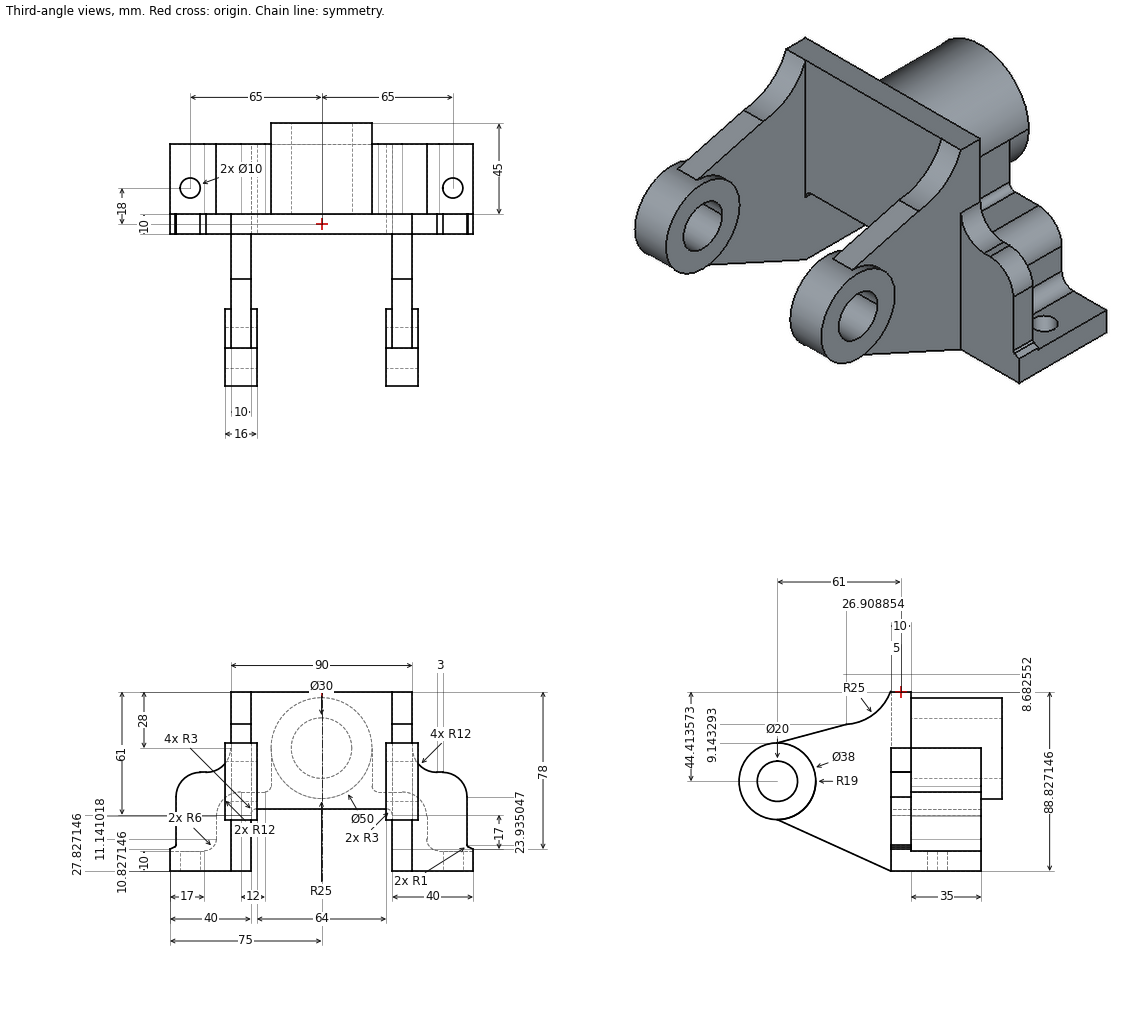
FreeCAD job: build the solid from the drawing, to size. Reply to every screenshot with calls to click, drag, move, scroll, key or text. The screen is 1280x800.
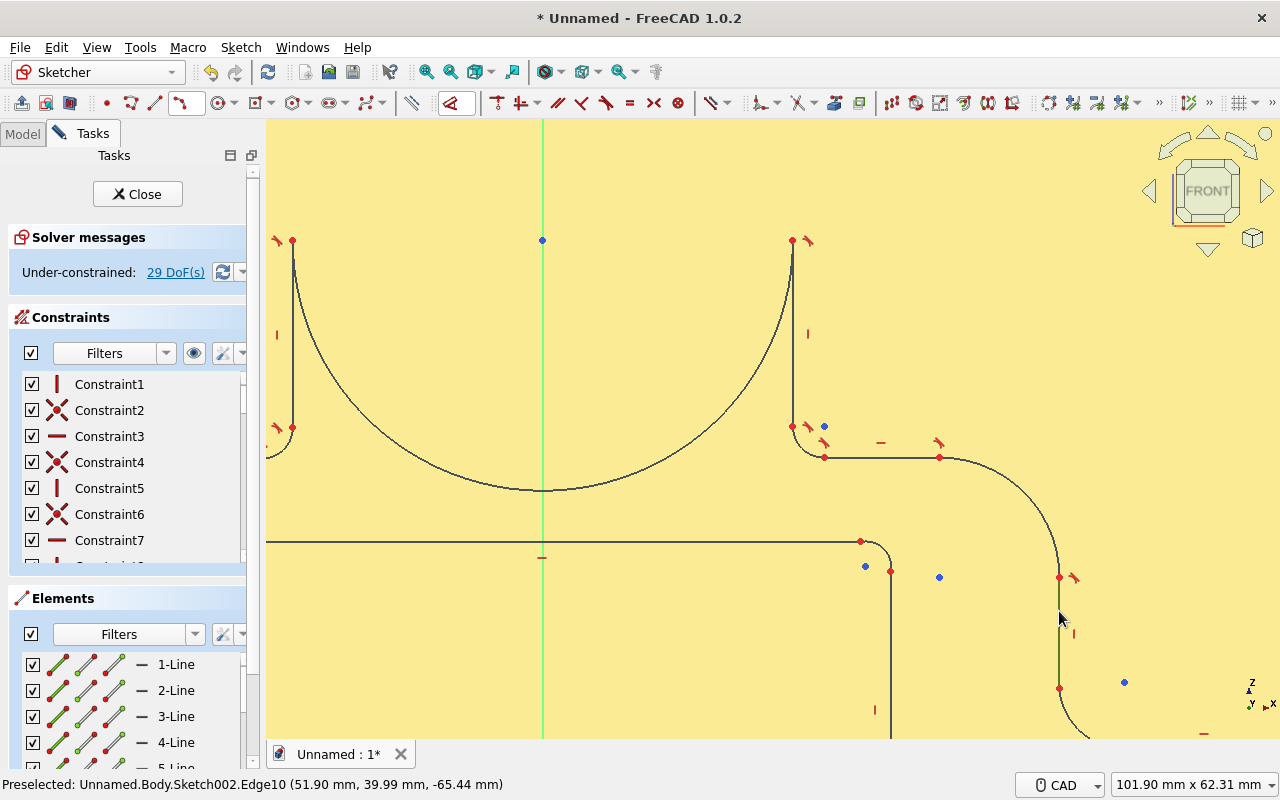
click(1063, 707)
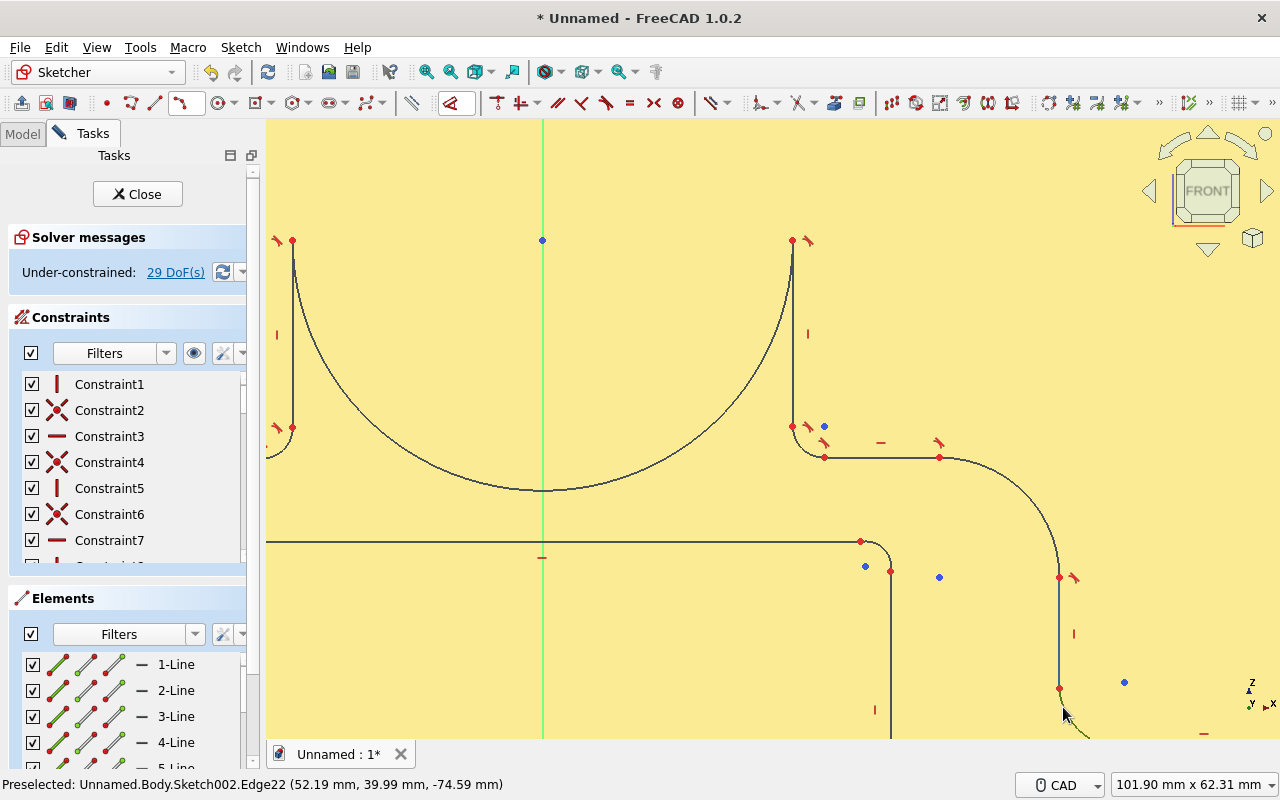
key(t)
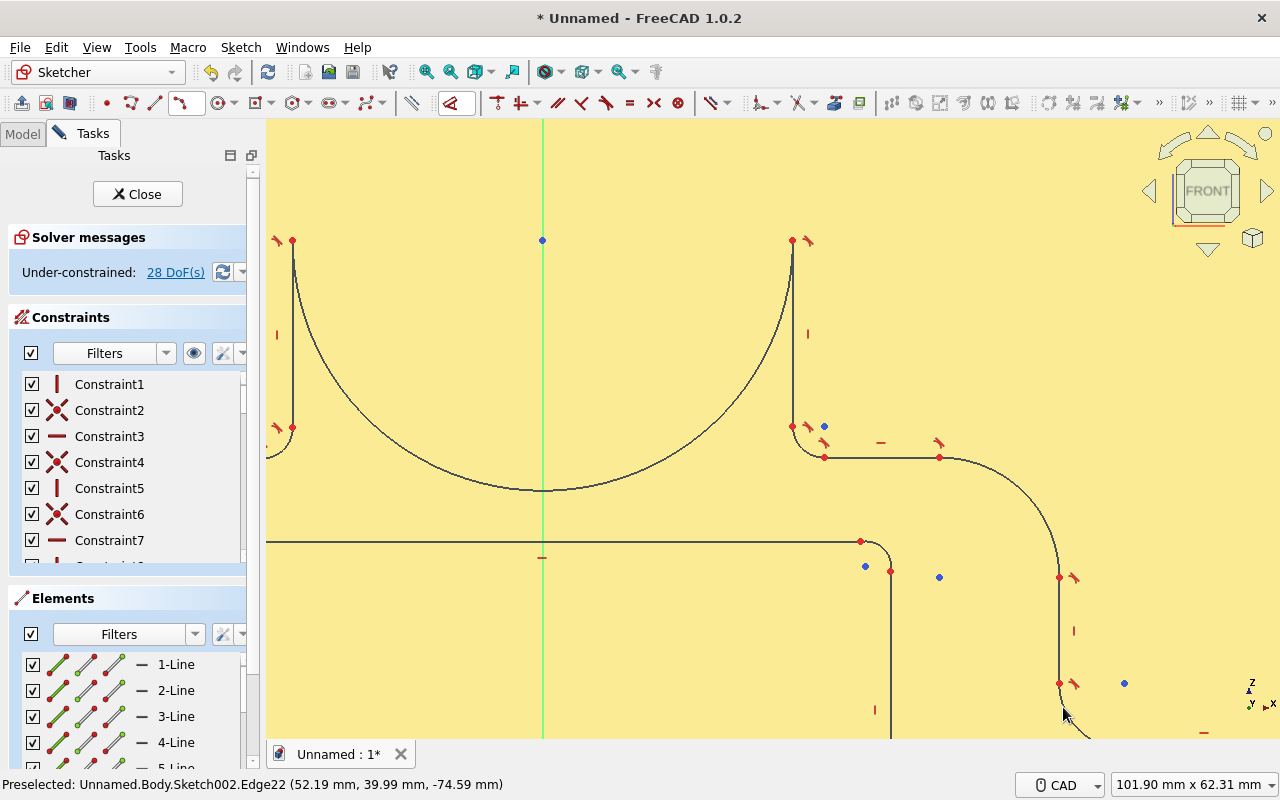
scroll(799, 444, down, 5)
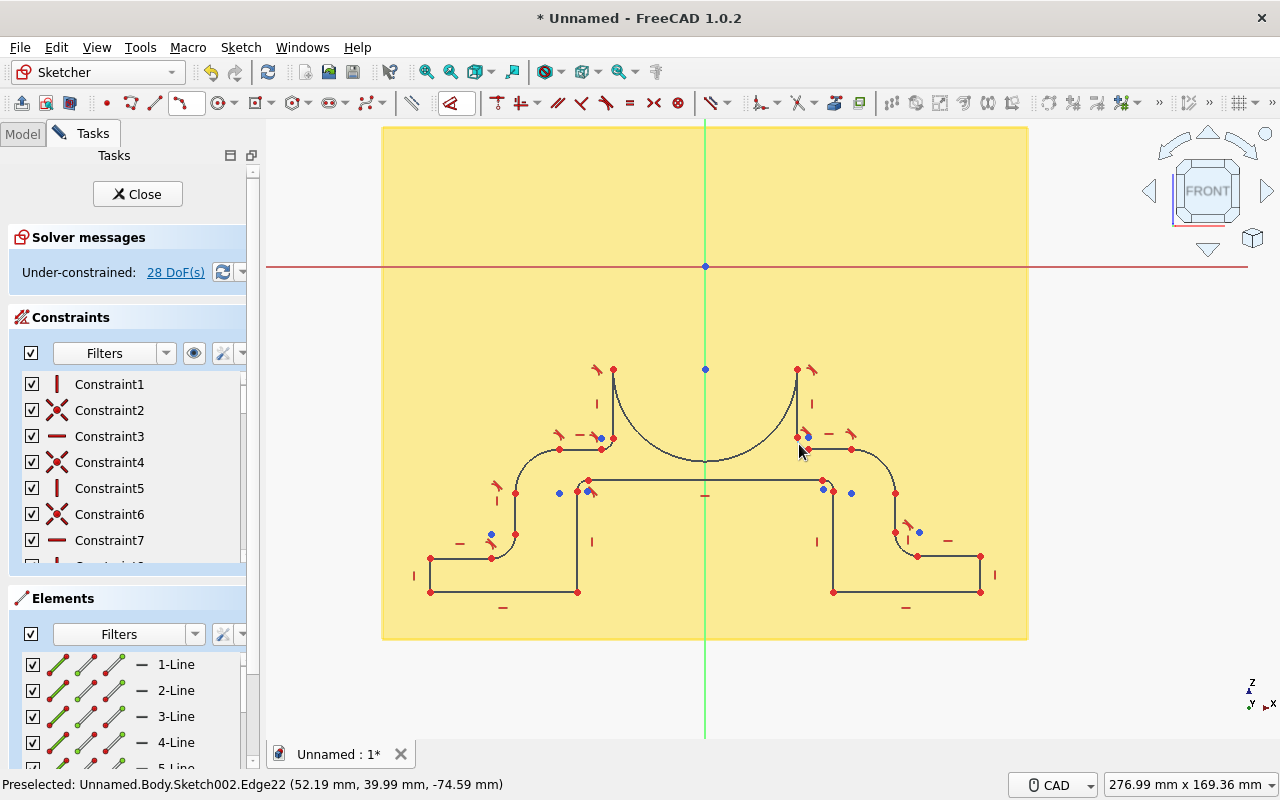
click(936, 556)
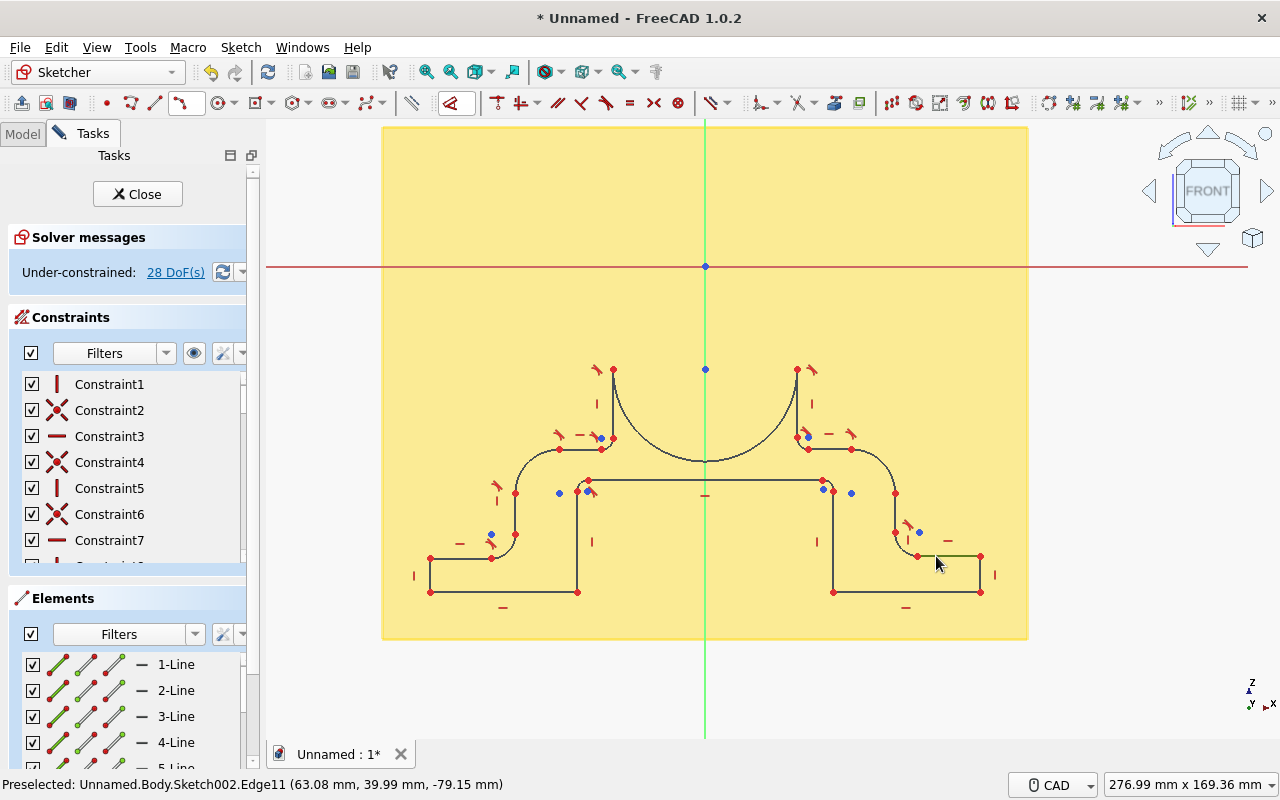
scroll(897, 543, up, 2)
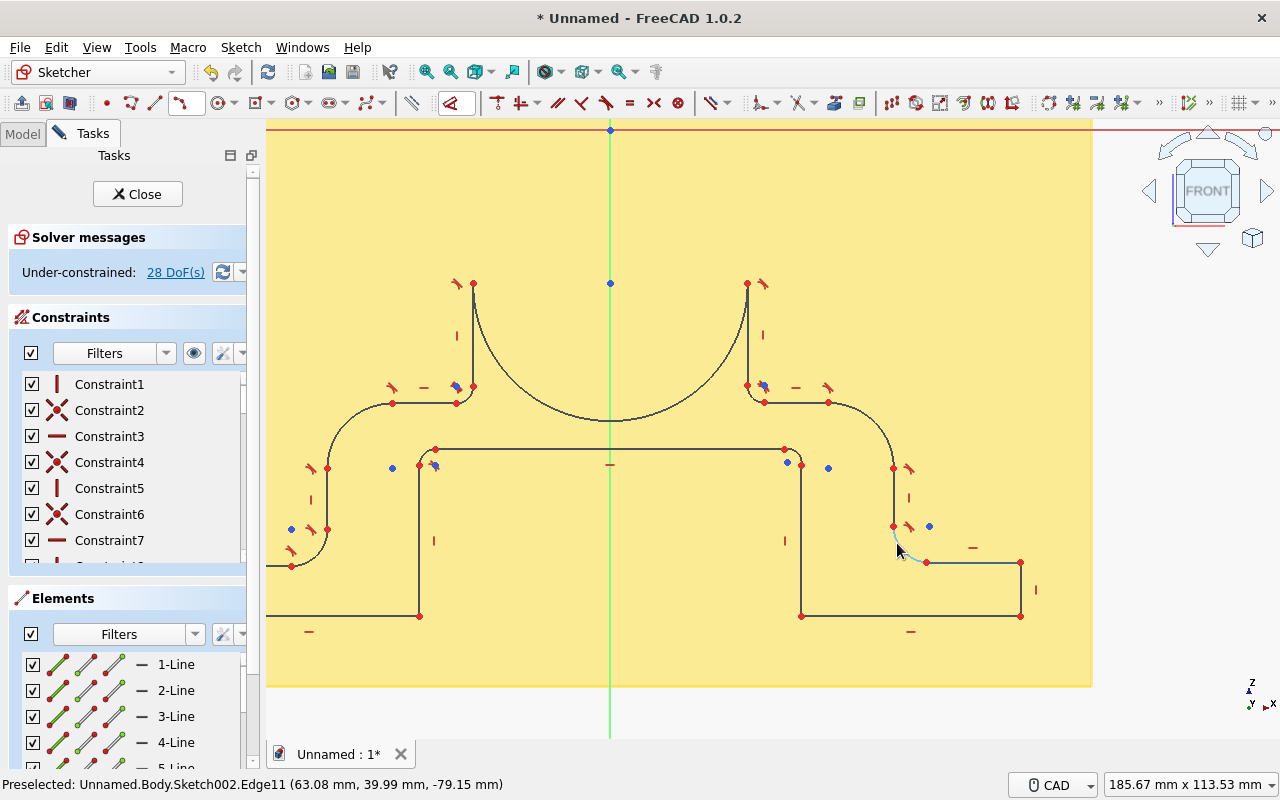
click(897, 542)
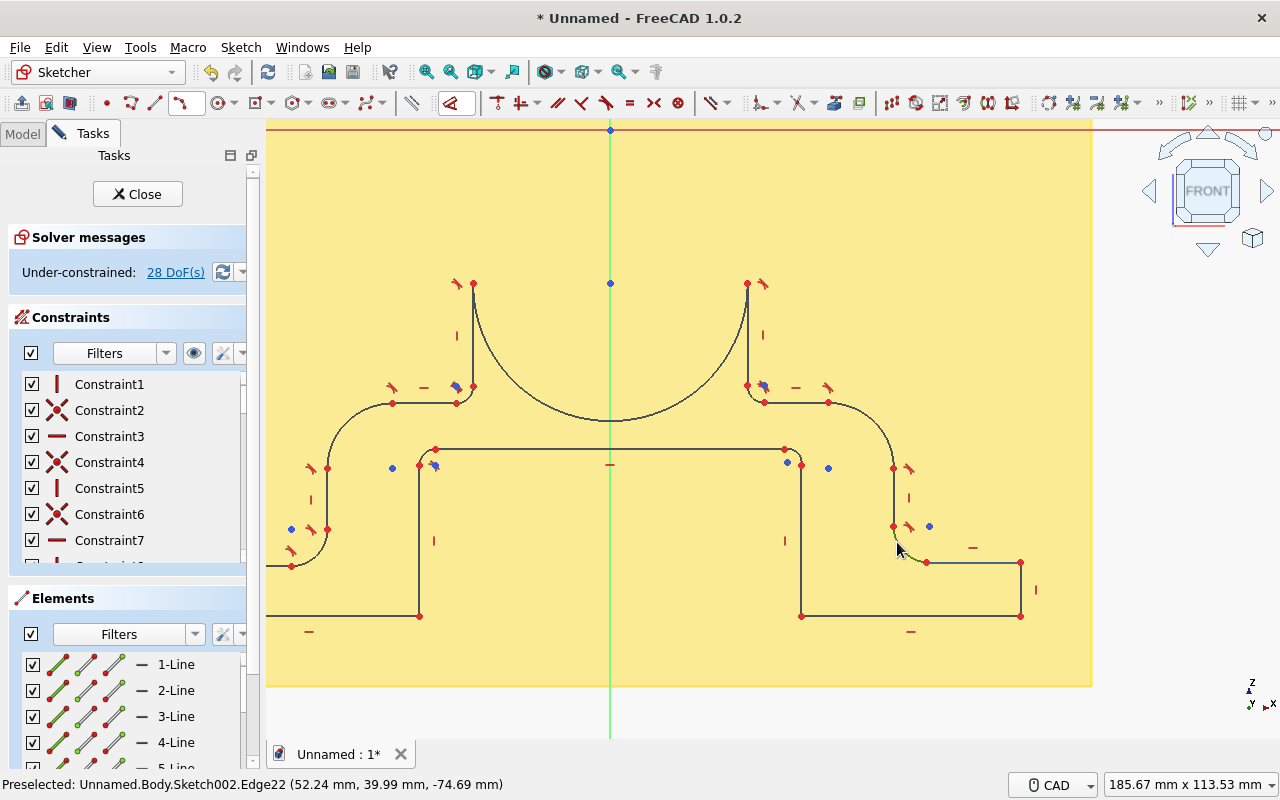
key(t)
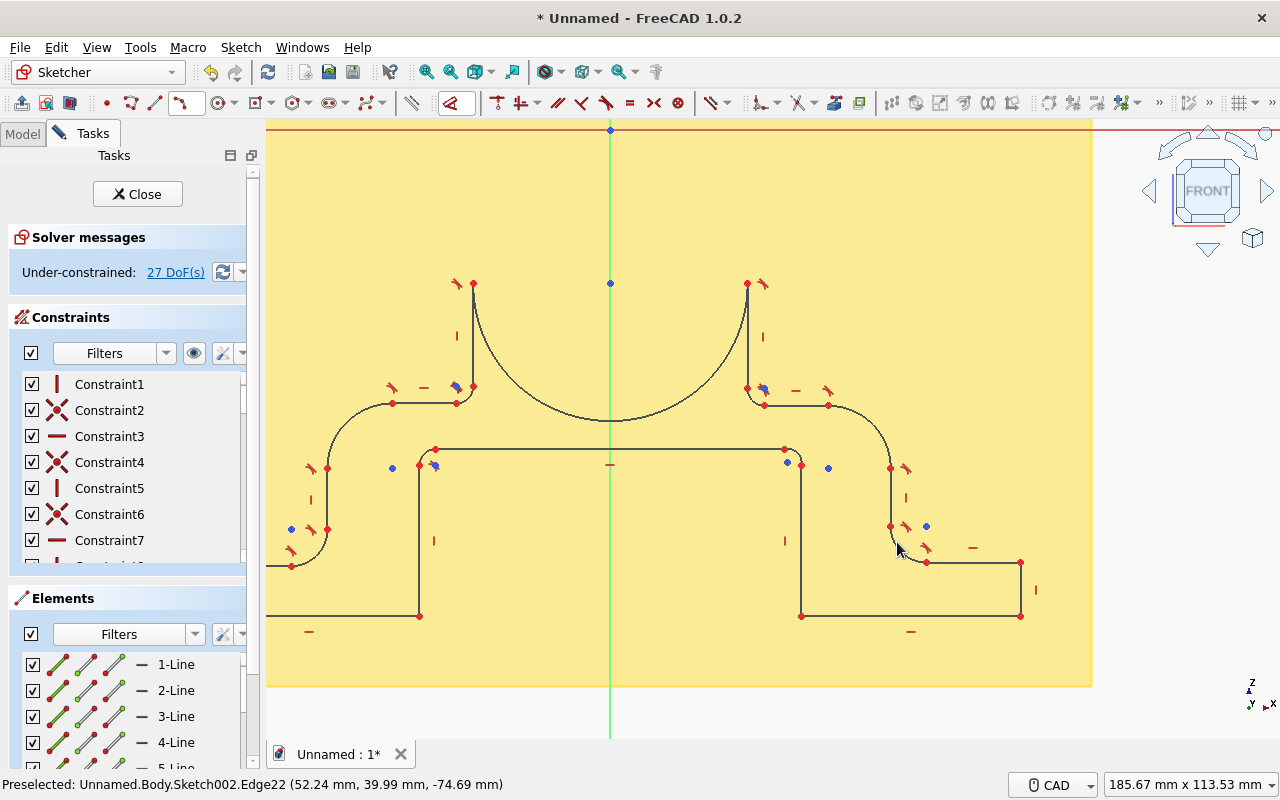
click(801, 571)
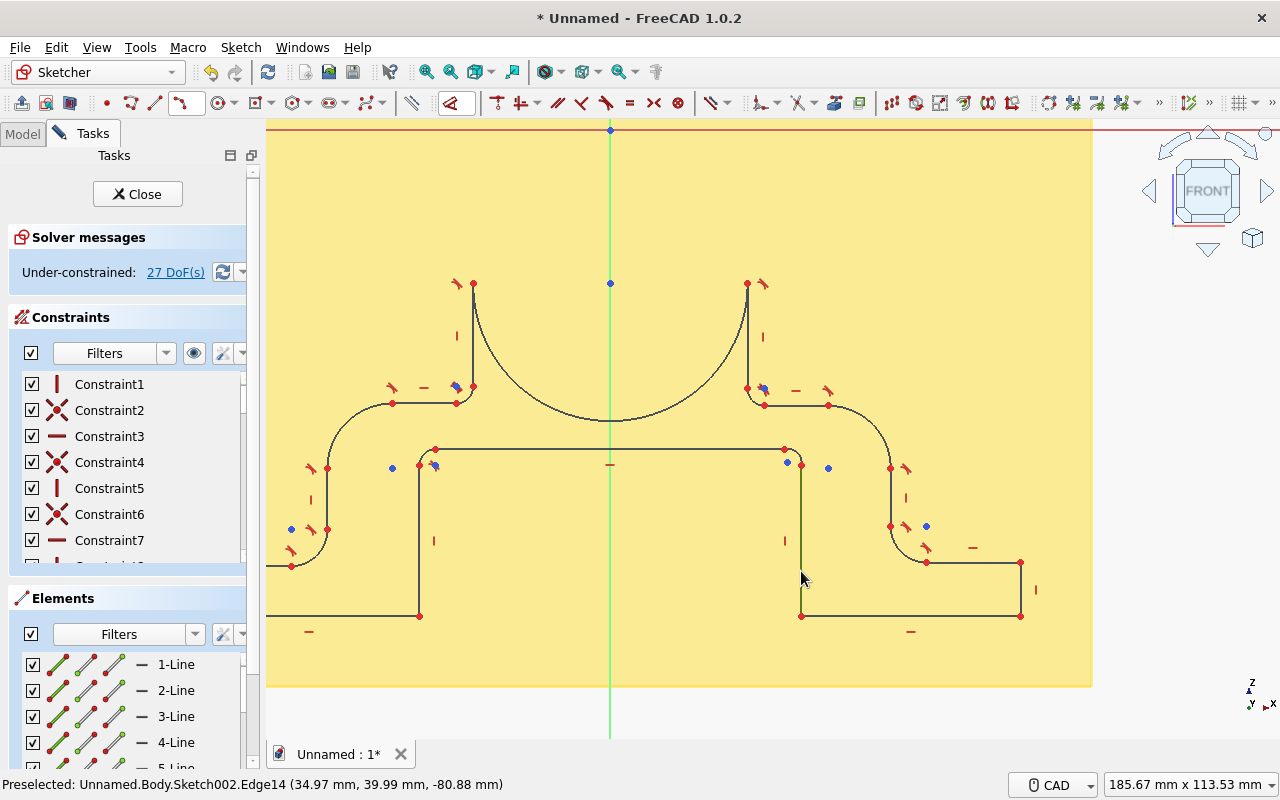
click(798, 453)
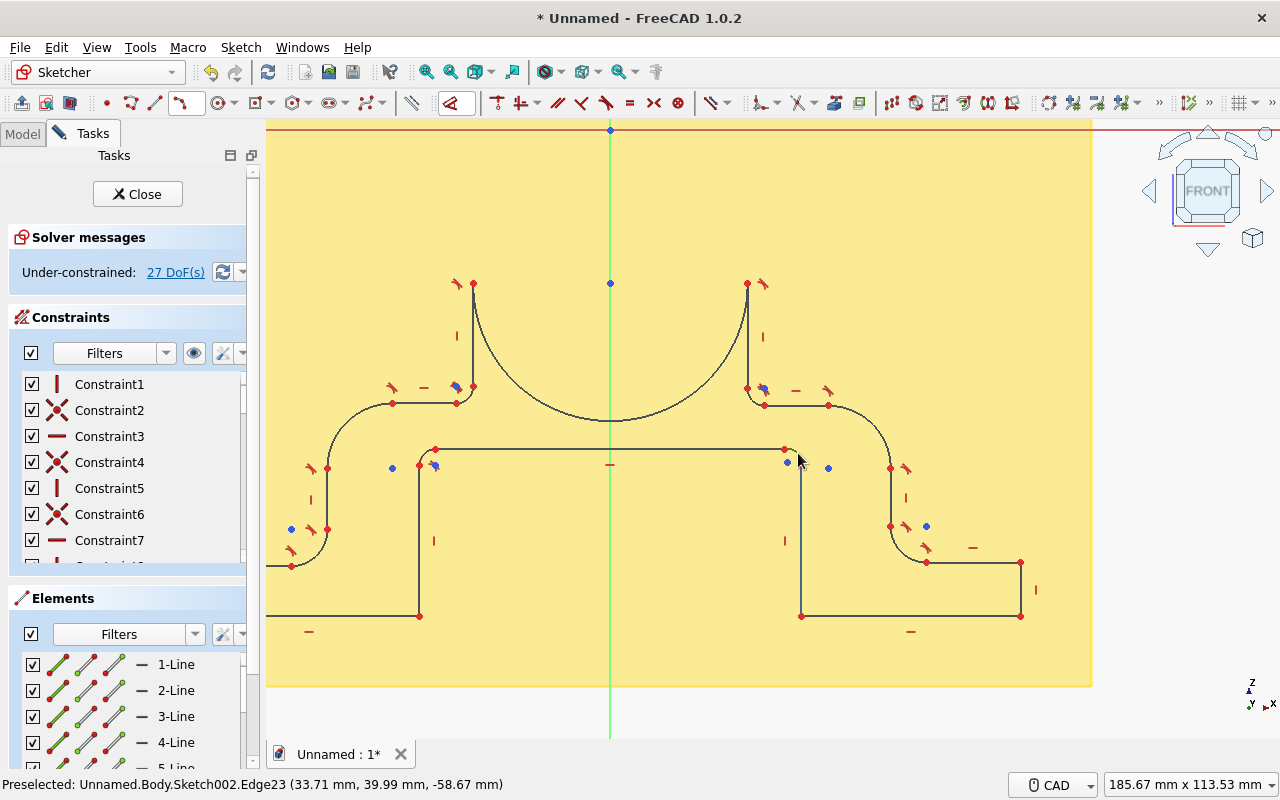
click(606, 104)